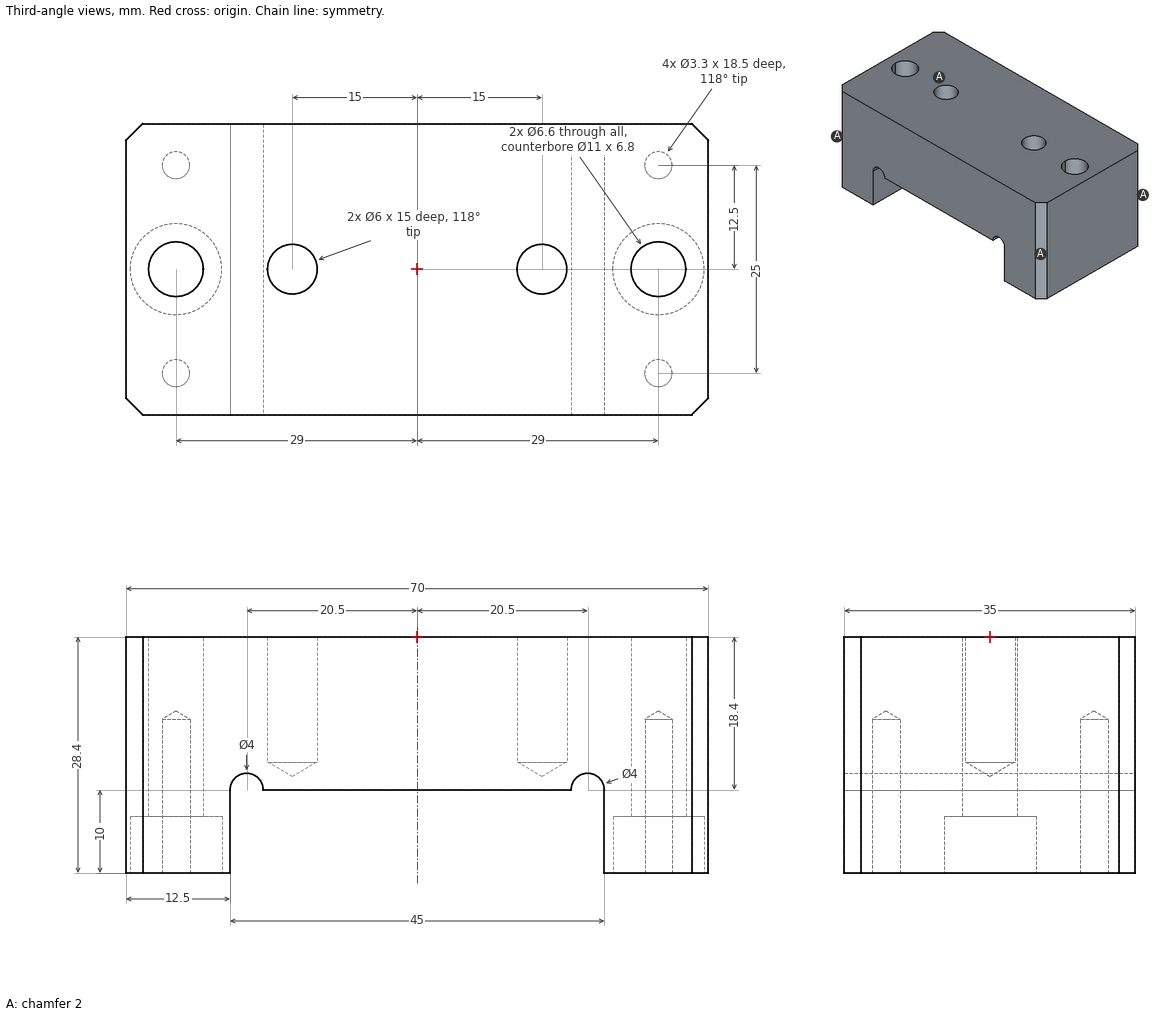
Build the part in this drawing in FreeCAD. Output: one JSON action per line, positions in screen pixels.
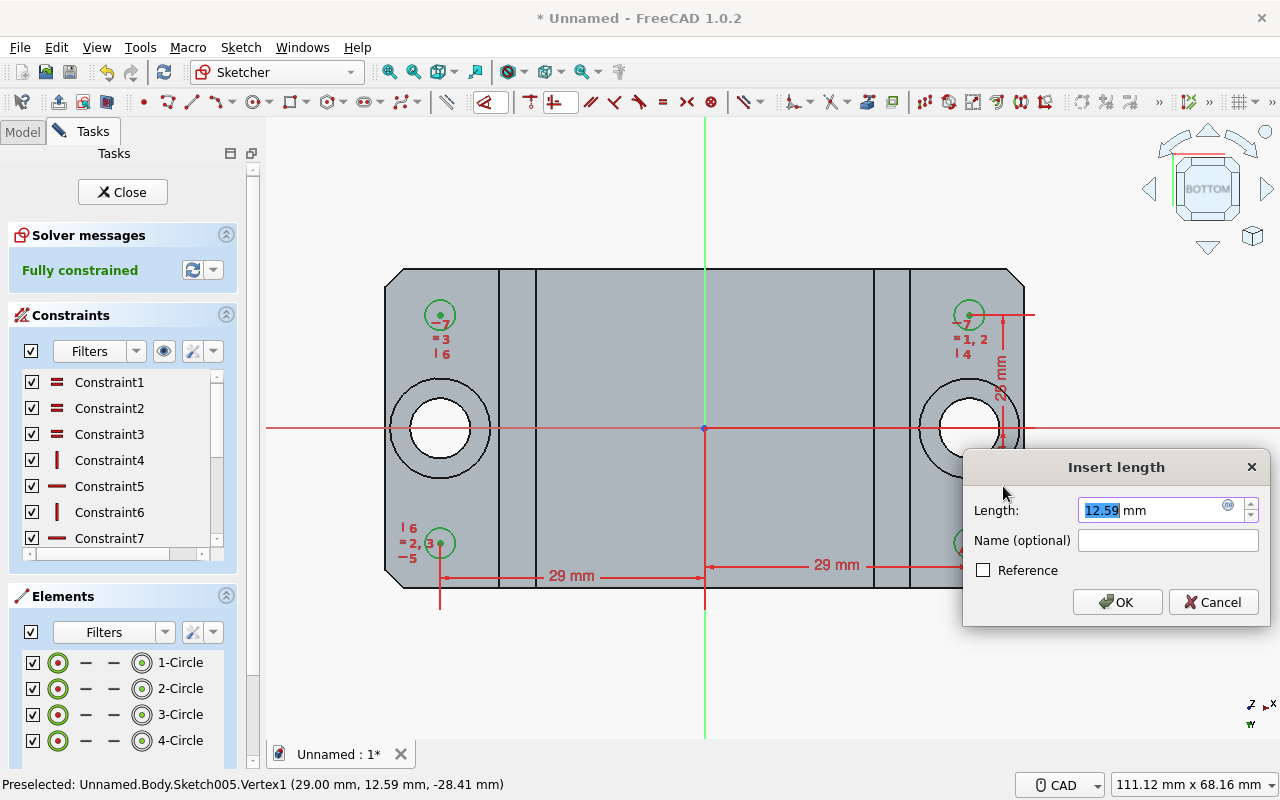
{"action": "type", "text": "12.5"}
{"action": "key", "text": "Return"}
{"action": "key", "text": "Escape"}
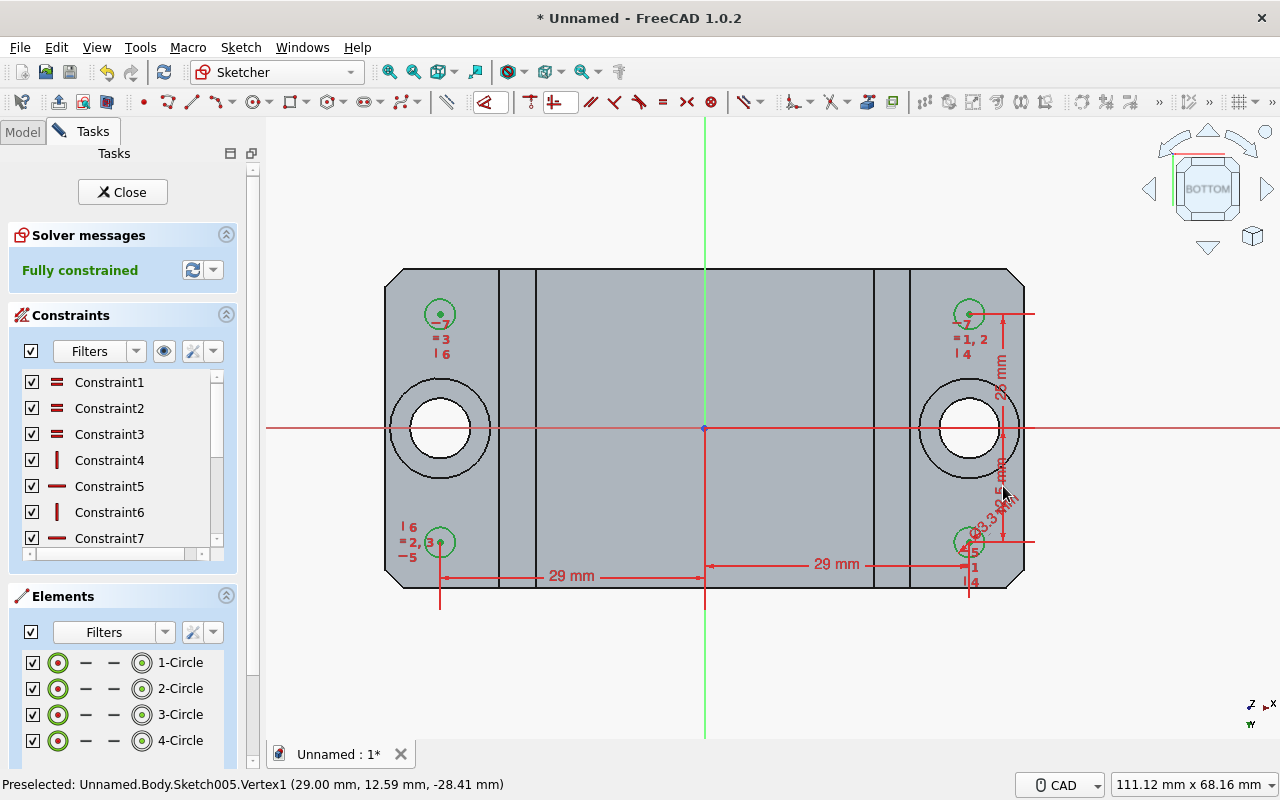
{"action": "left_click", "coordinate": [123, 192]}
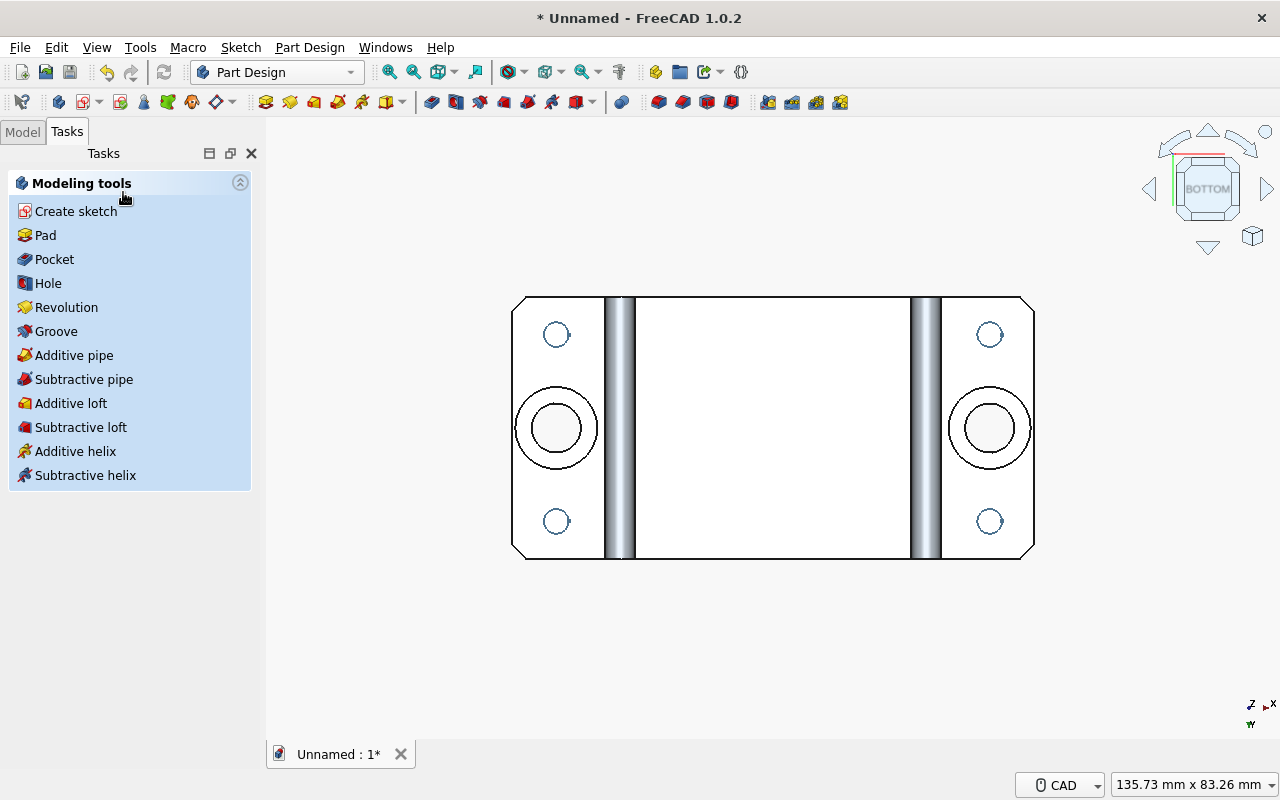
{"action": "left_click", "coordinate": [456, 102]}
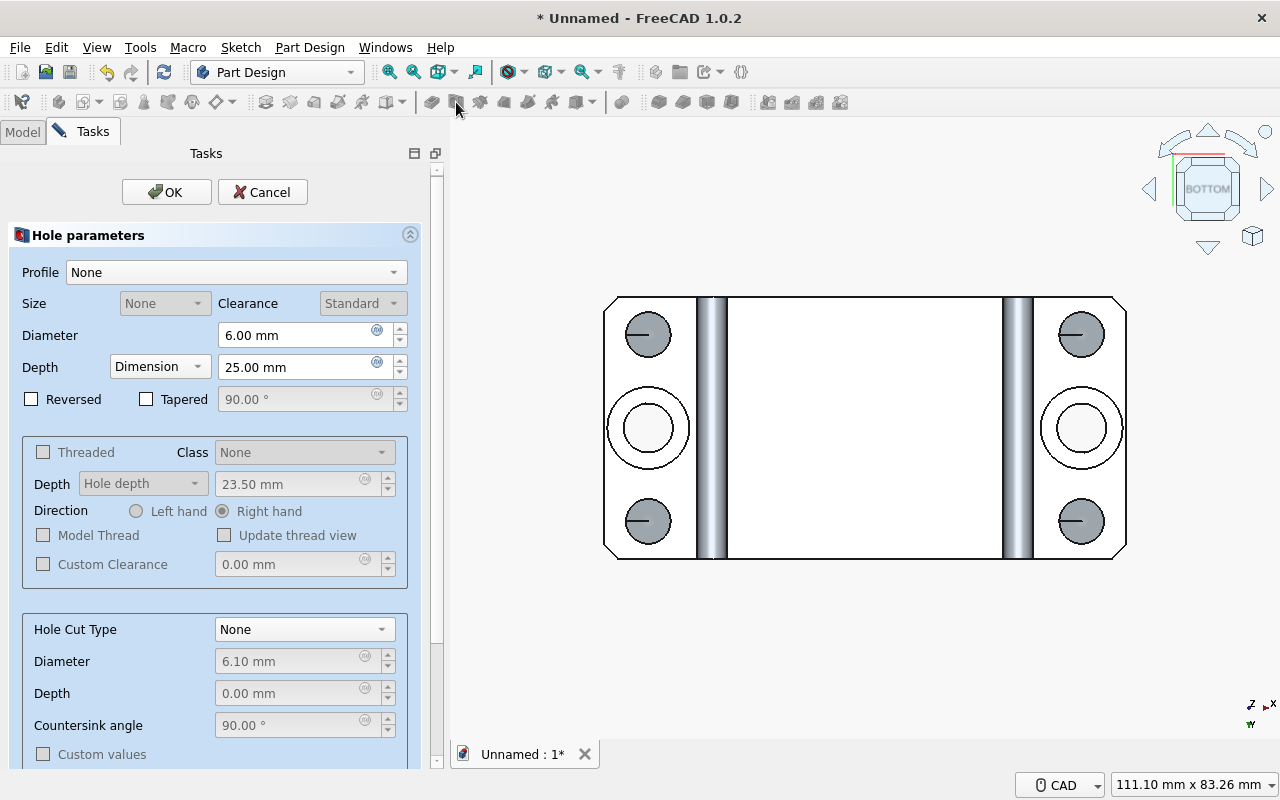
{"action": "triple_click", "coordinate": [305, 335]}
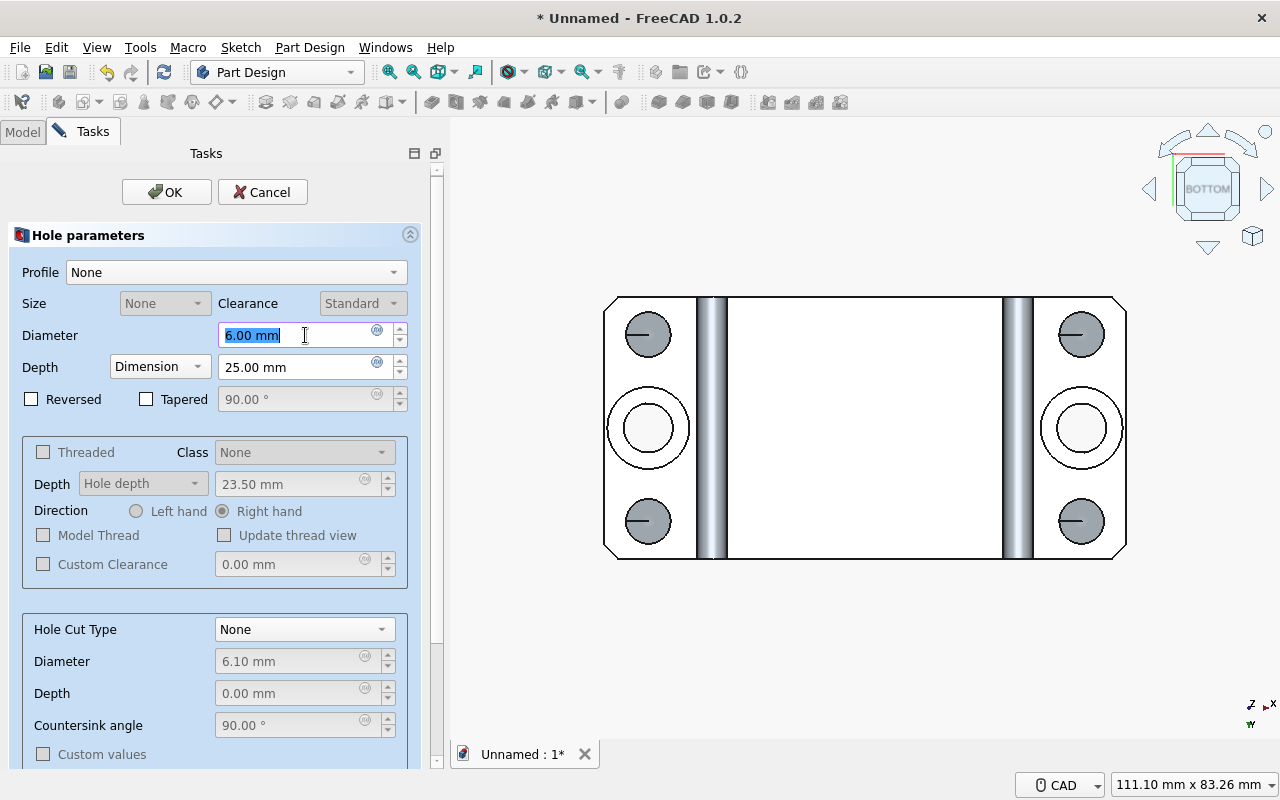
{"action": "type", "text": "3.3"}
{"action": "key", "text": "Tab"}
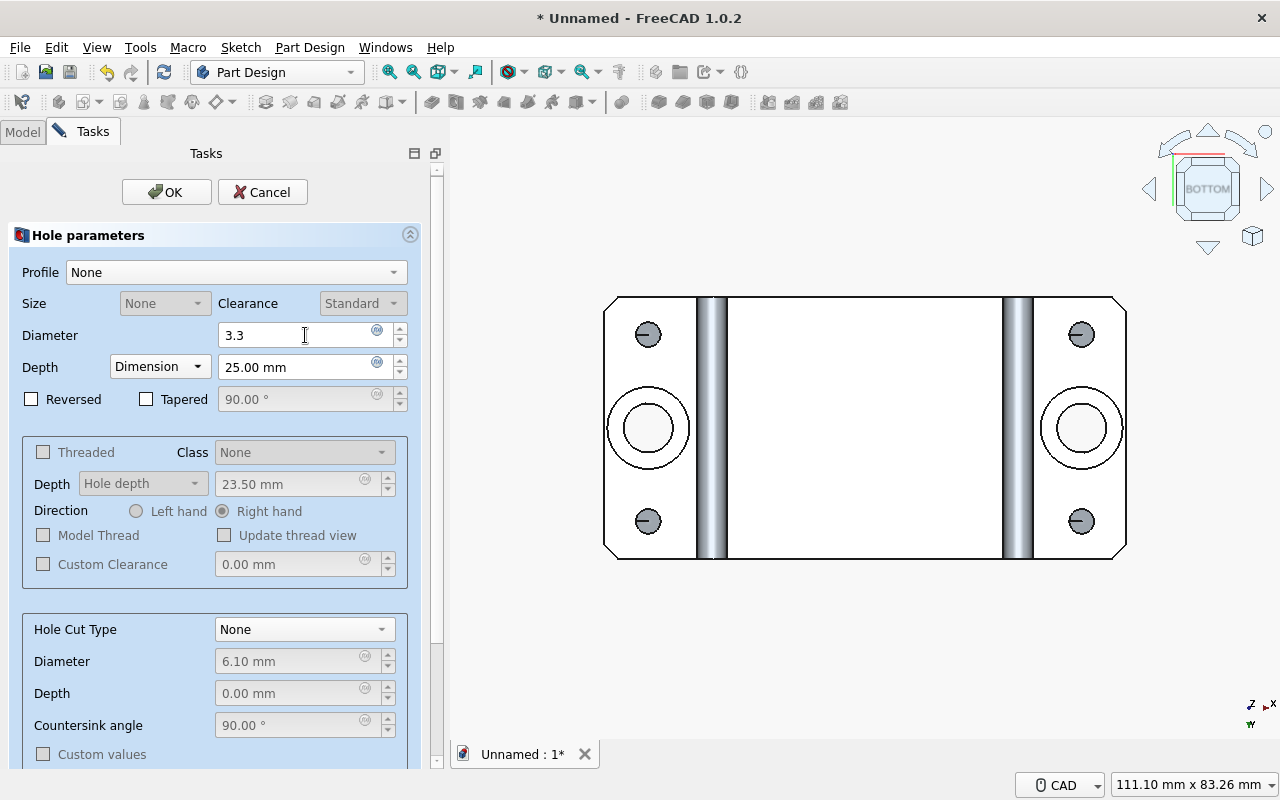
{"action": "triple_click", "coordinate": [305, 367]}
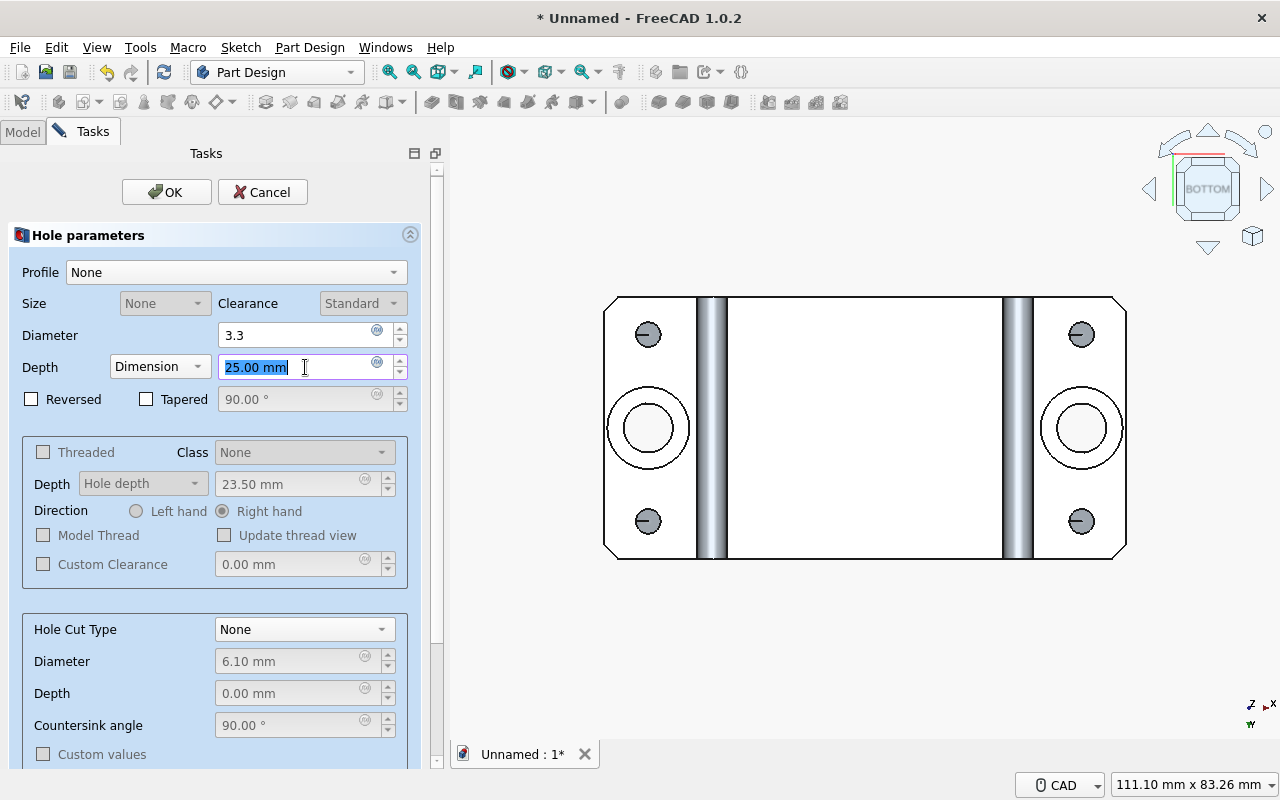
{"action": "type", "text": "18.5"}
{"action": "key", "text": "Tab"}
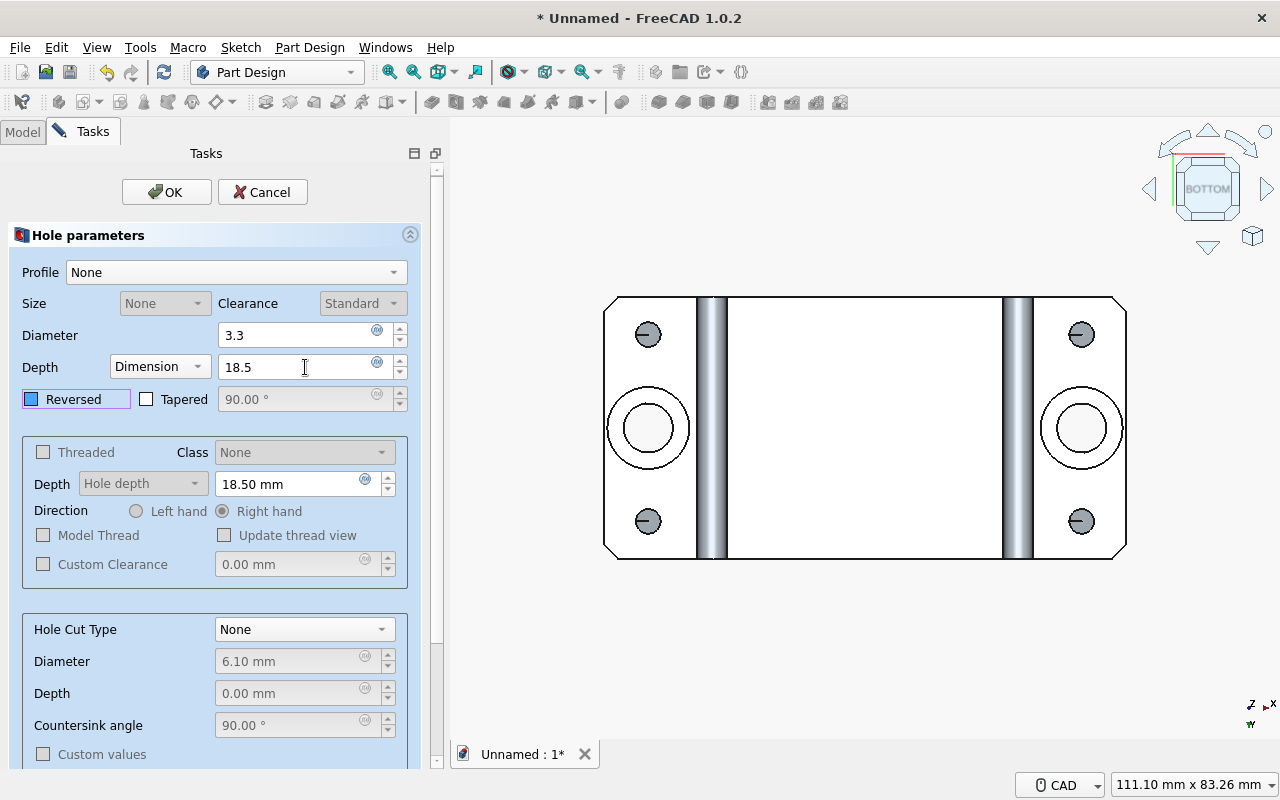
{"action": "left_click", "coordinate": [167, 192]}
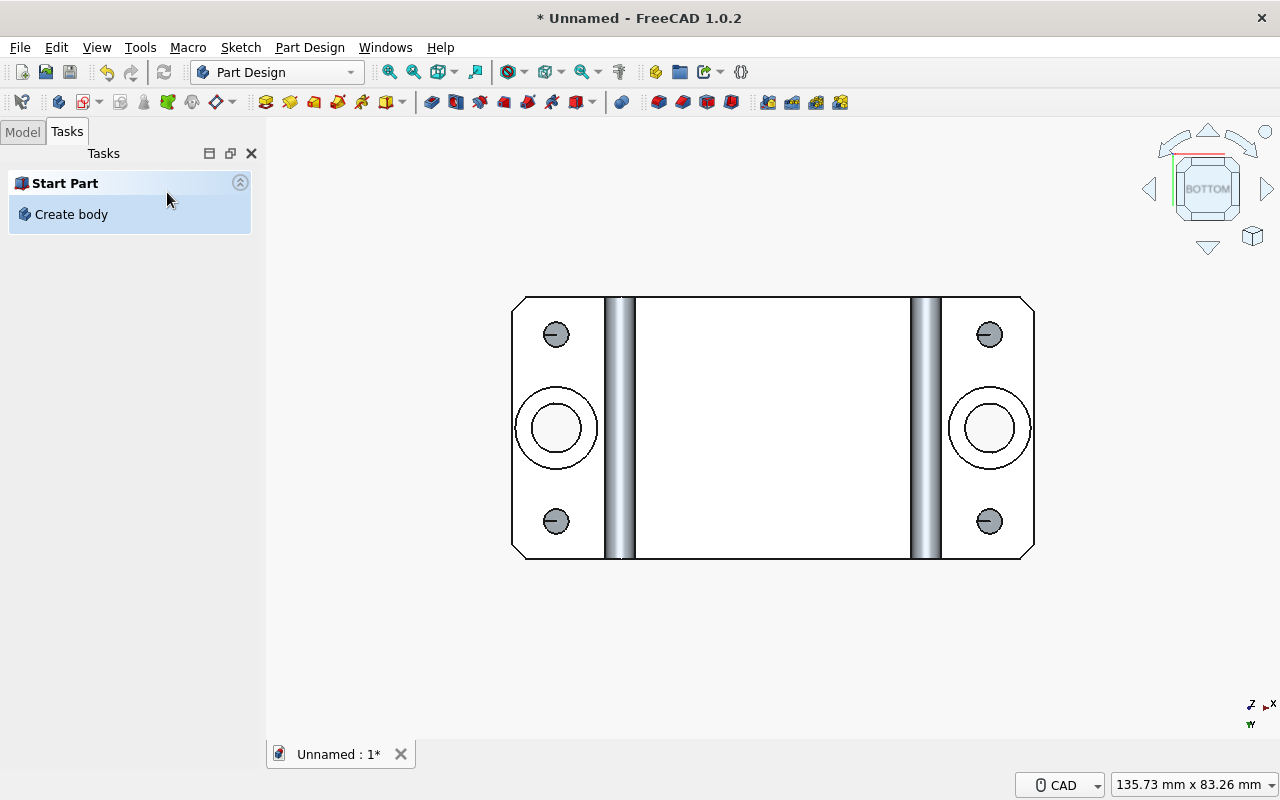
{"action": "key", "text": "0"}